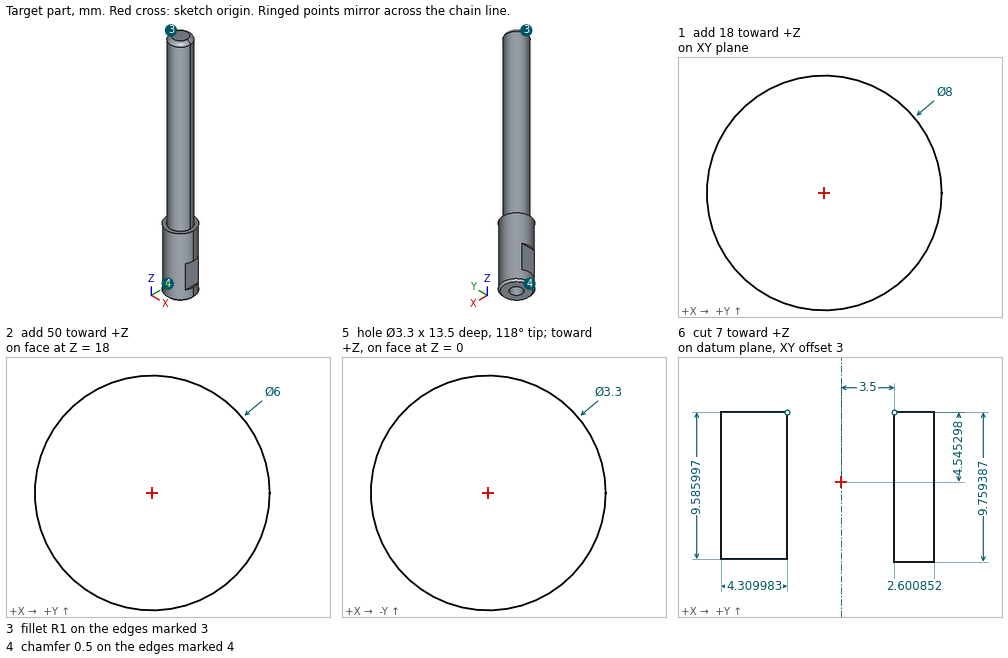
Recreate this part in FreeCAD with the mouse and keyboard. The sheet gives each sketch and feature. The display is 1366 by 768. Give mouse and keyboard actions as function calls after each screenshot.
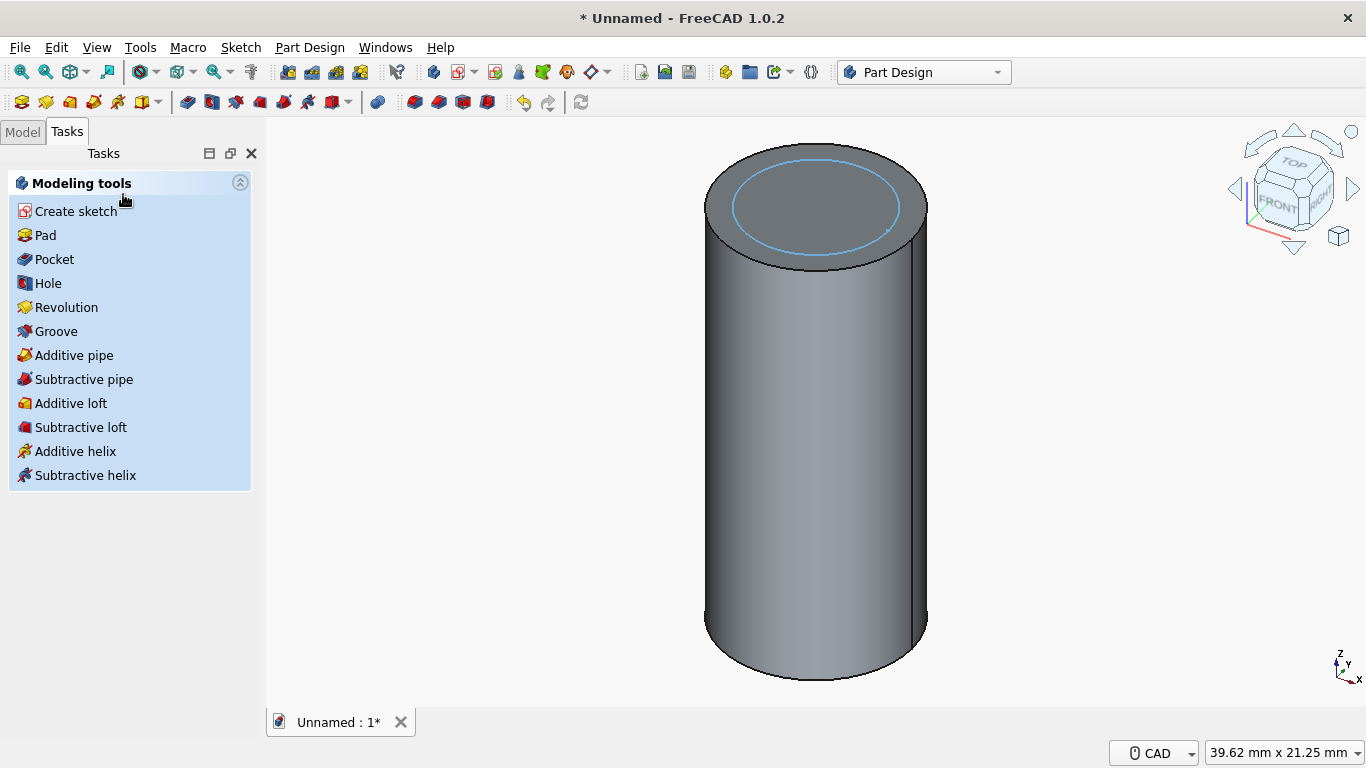
click(22, 102)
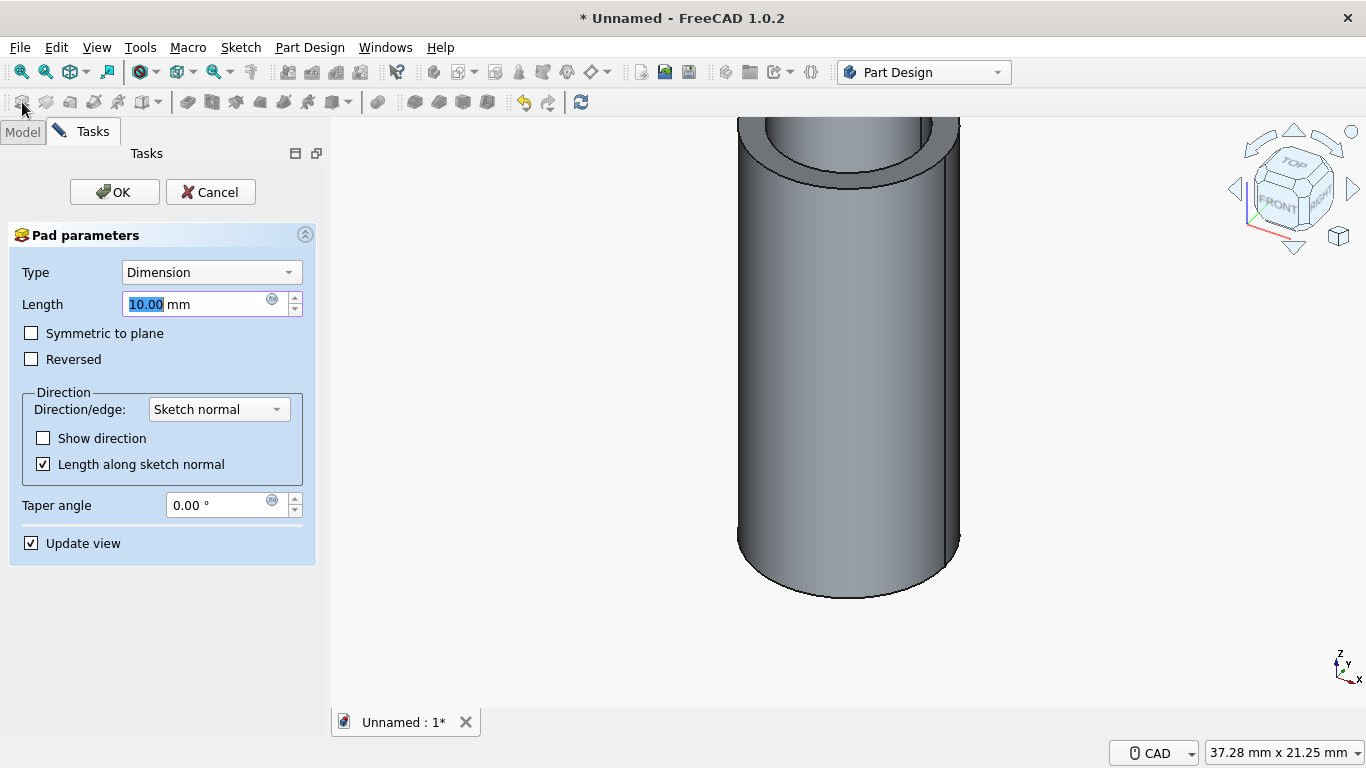
text(50)
key(Tab)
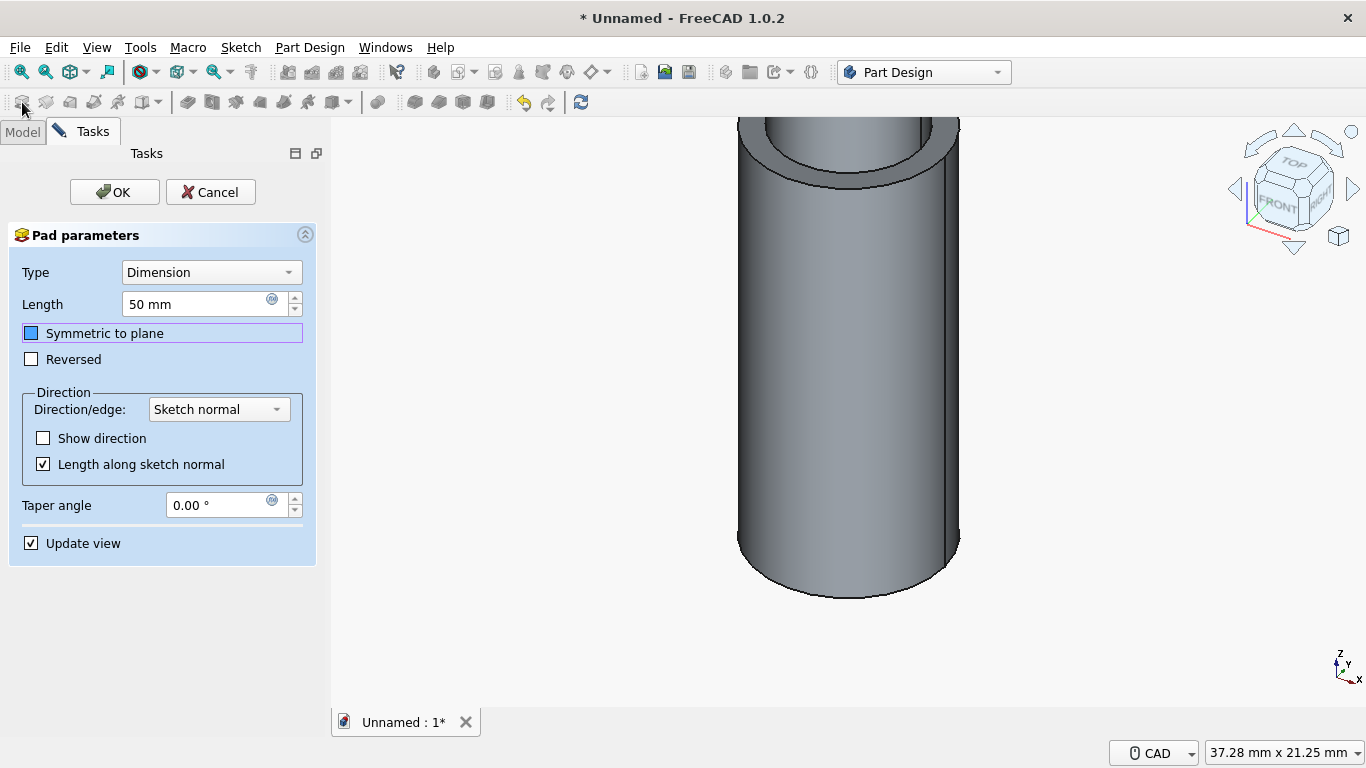
click(115, 192)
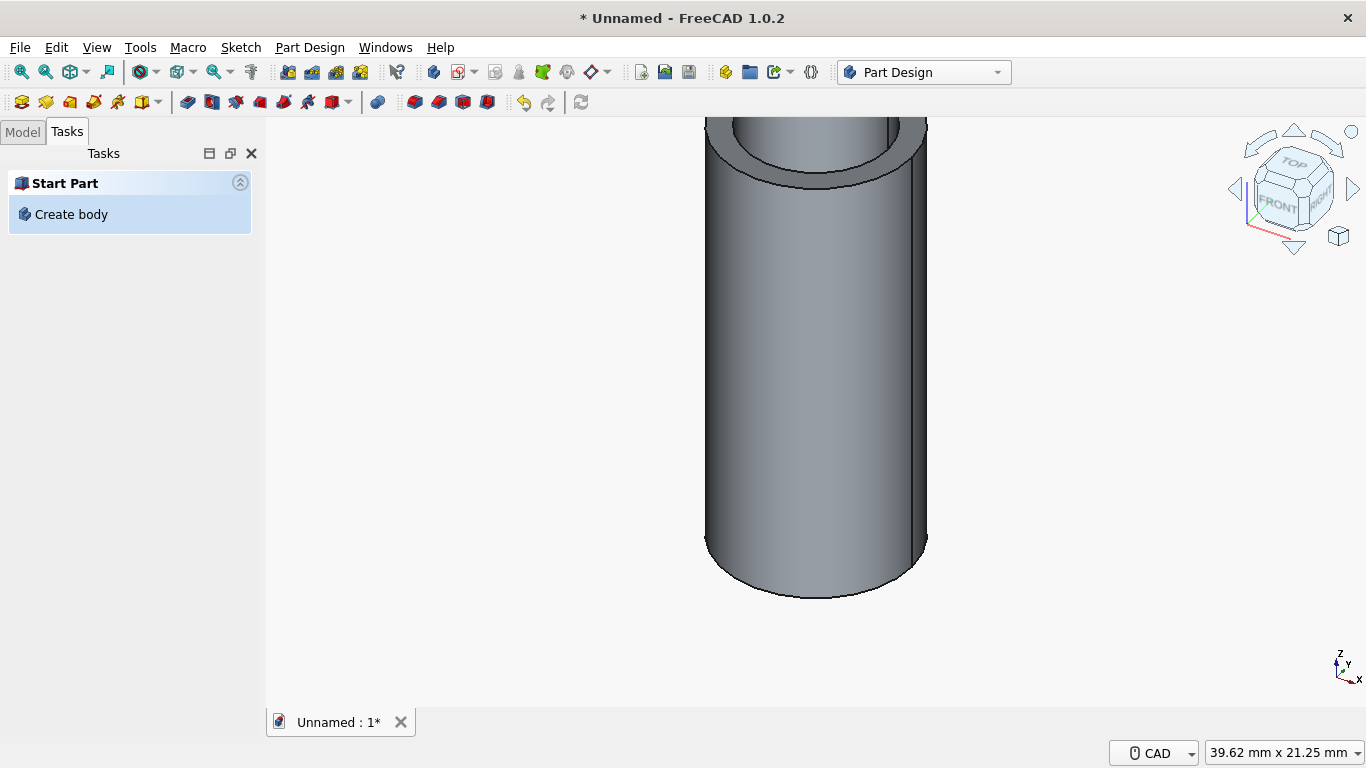
click(22, 72)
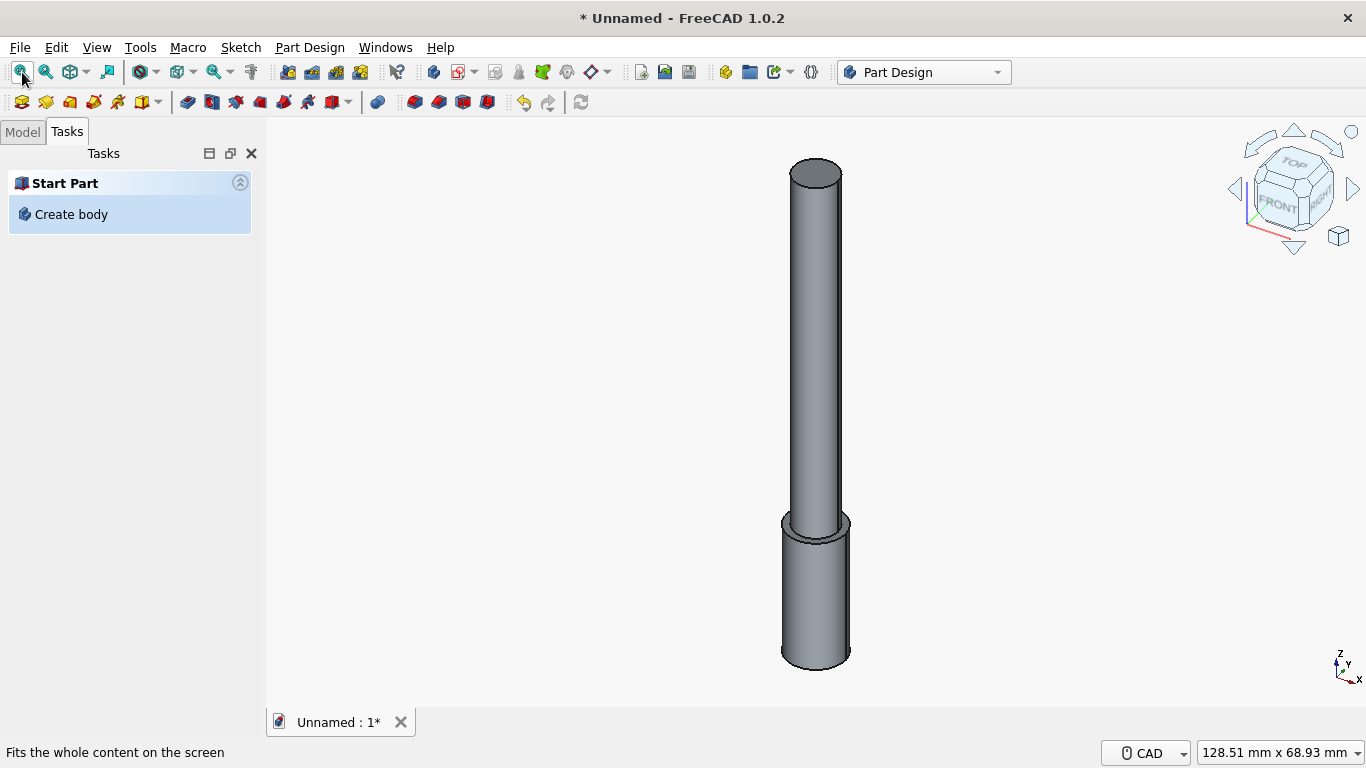
click(805, 159)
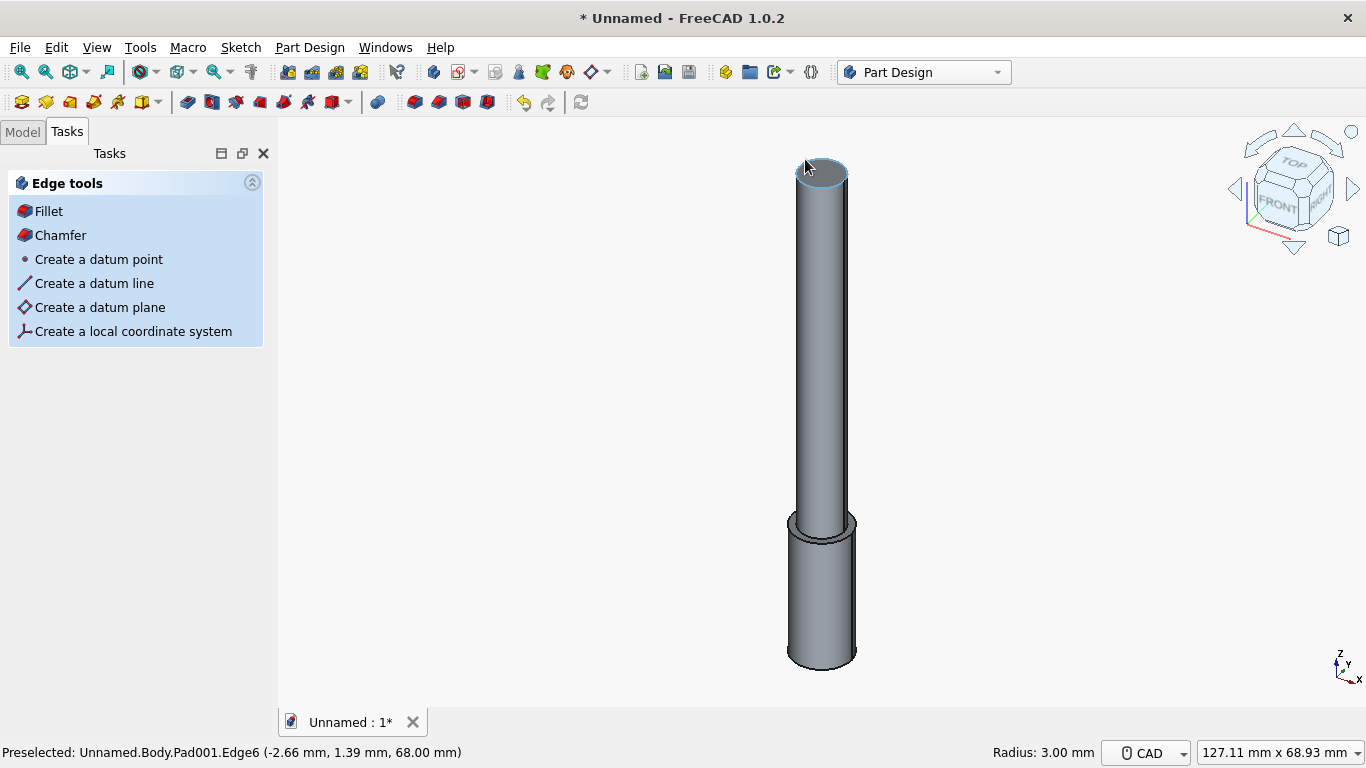
click(416, 102)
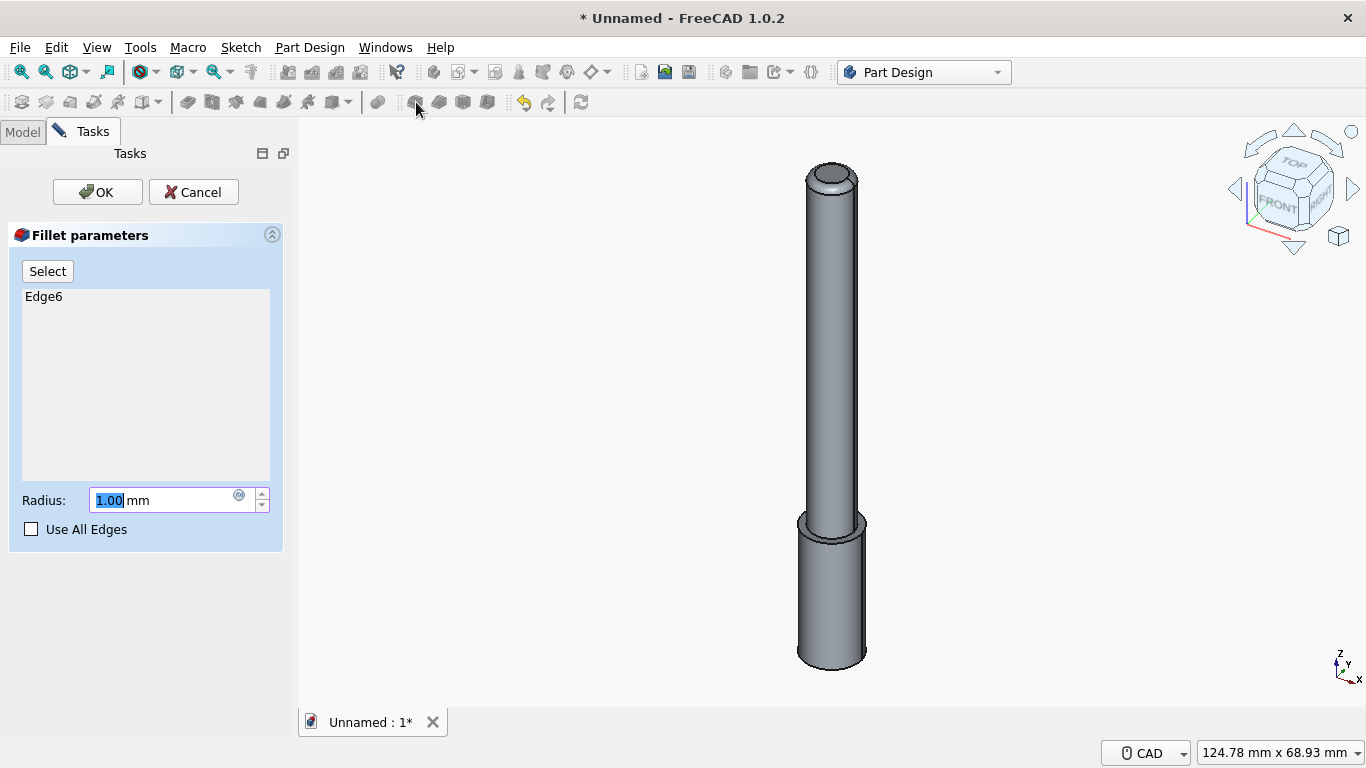
text(1)
key(Tab)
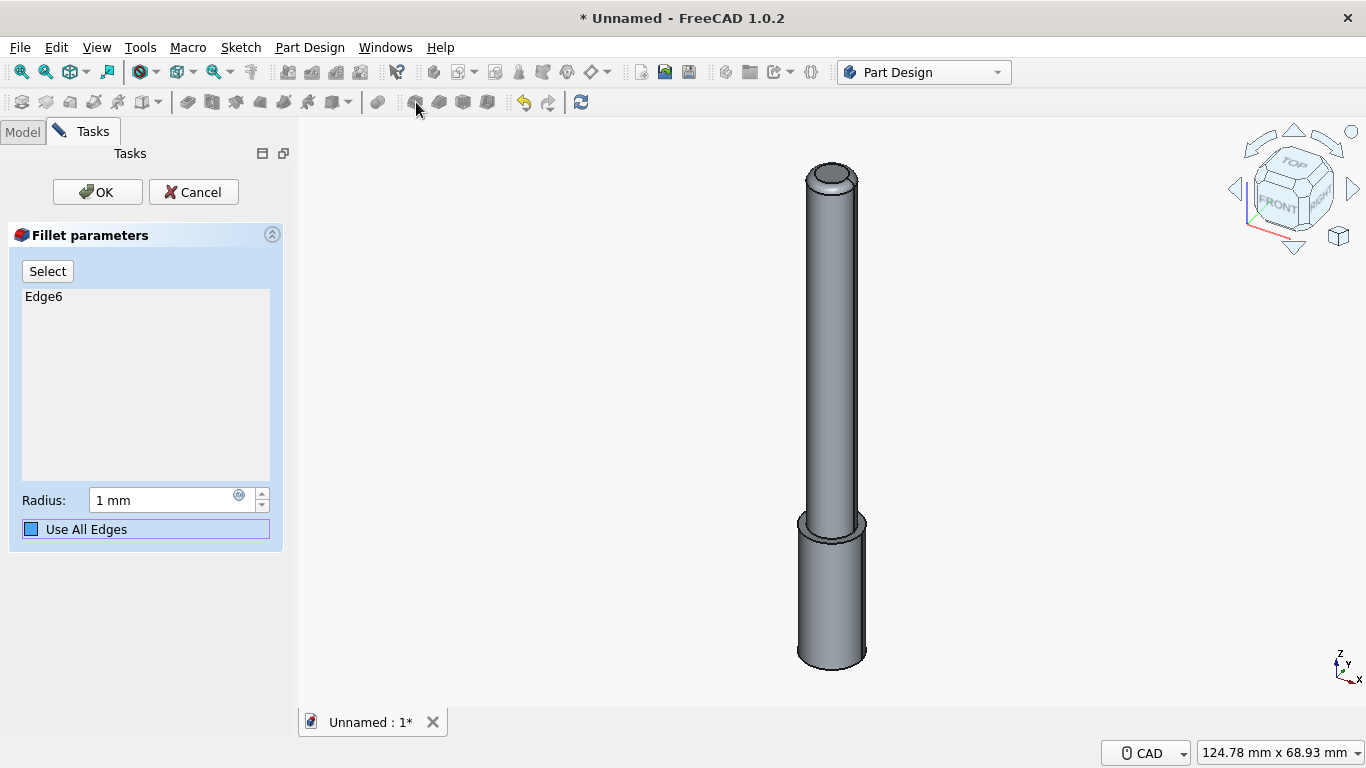
click(98, 192)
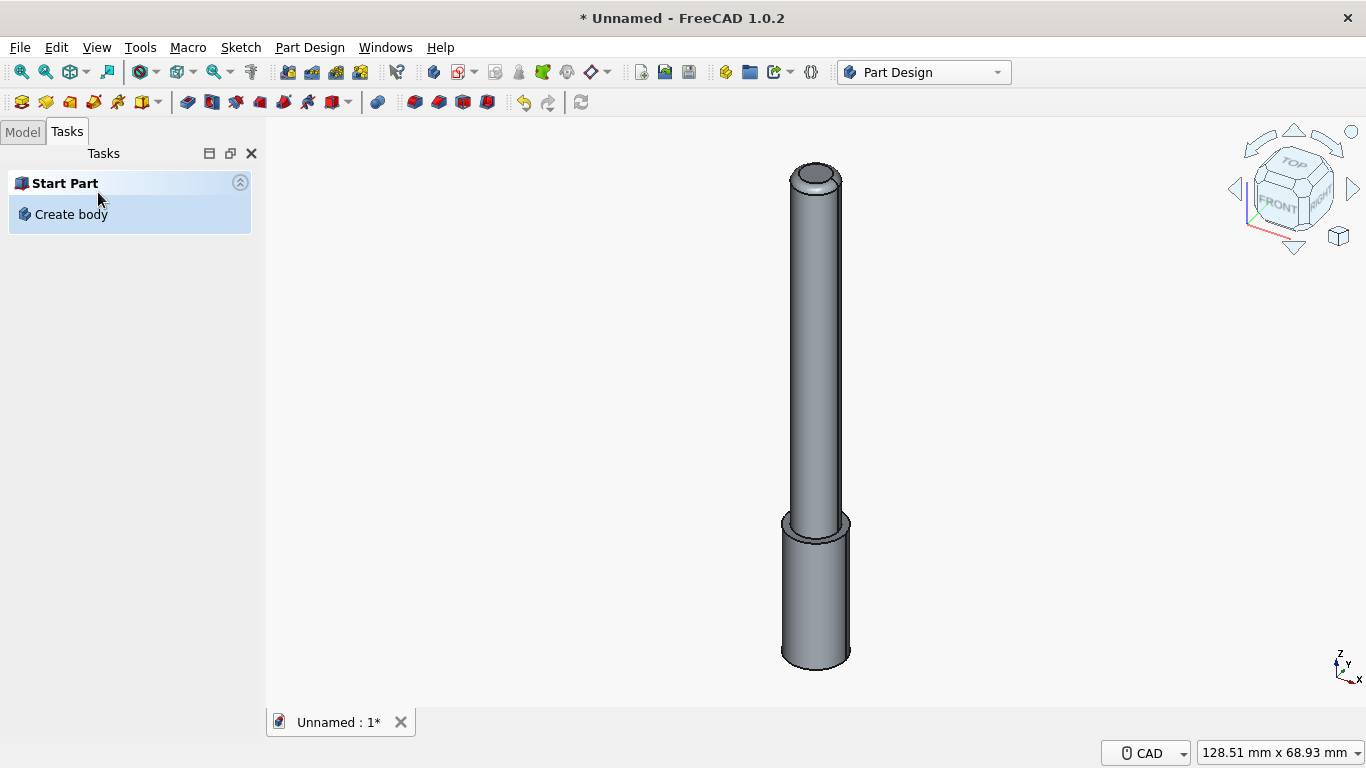
key(0)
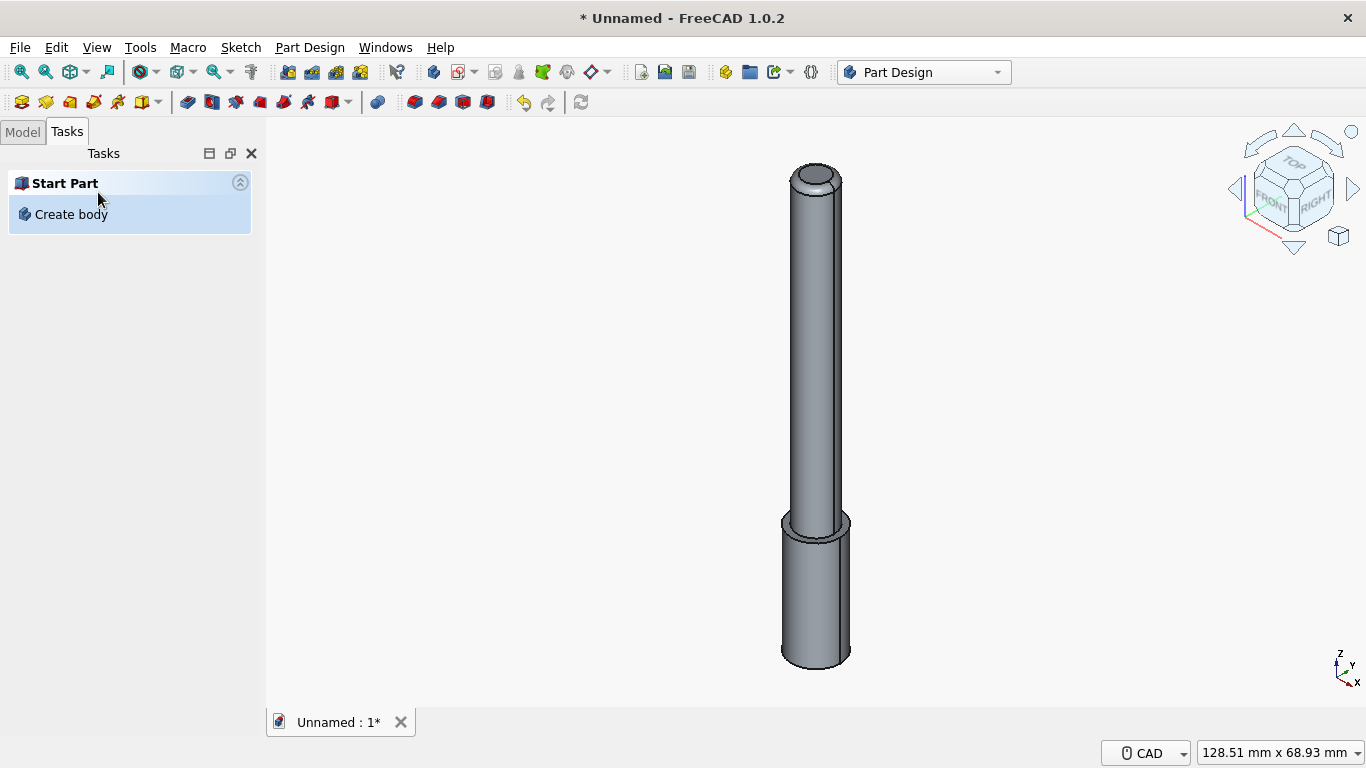
click(800, 666)